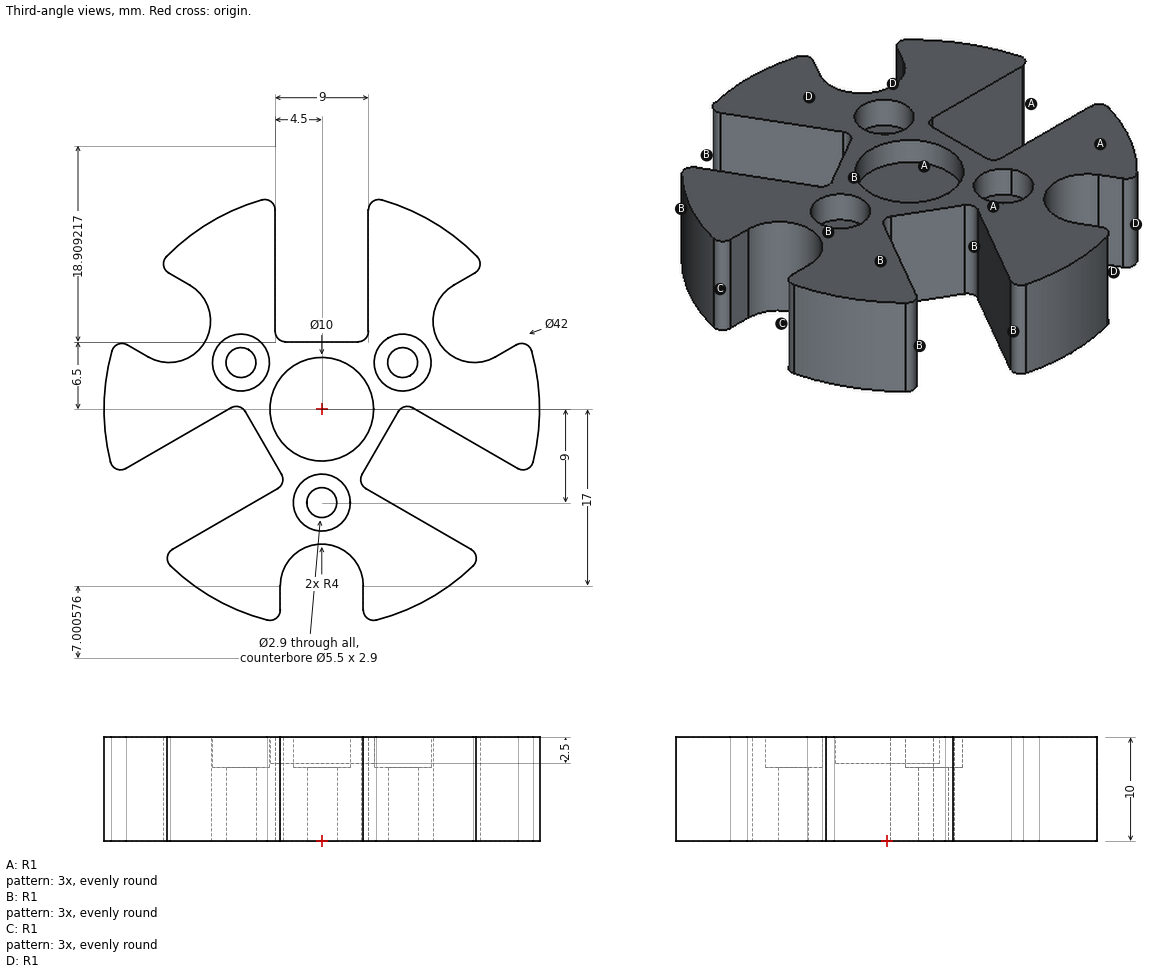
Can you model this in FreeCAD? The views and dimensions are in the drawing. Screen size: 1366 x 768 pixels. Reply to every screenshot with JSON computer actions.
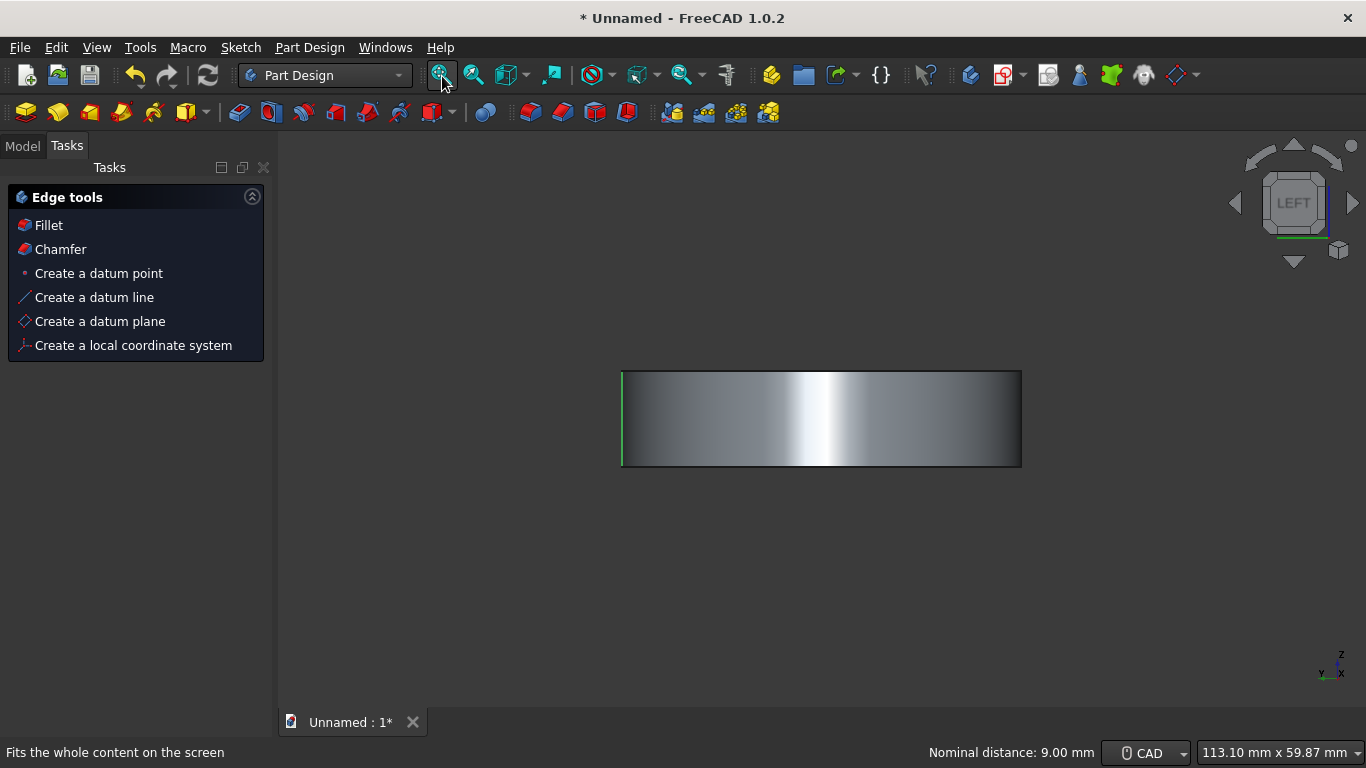
{"action": "key", "text": "v 3"}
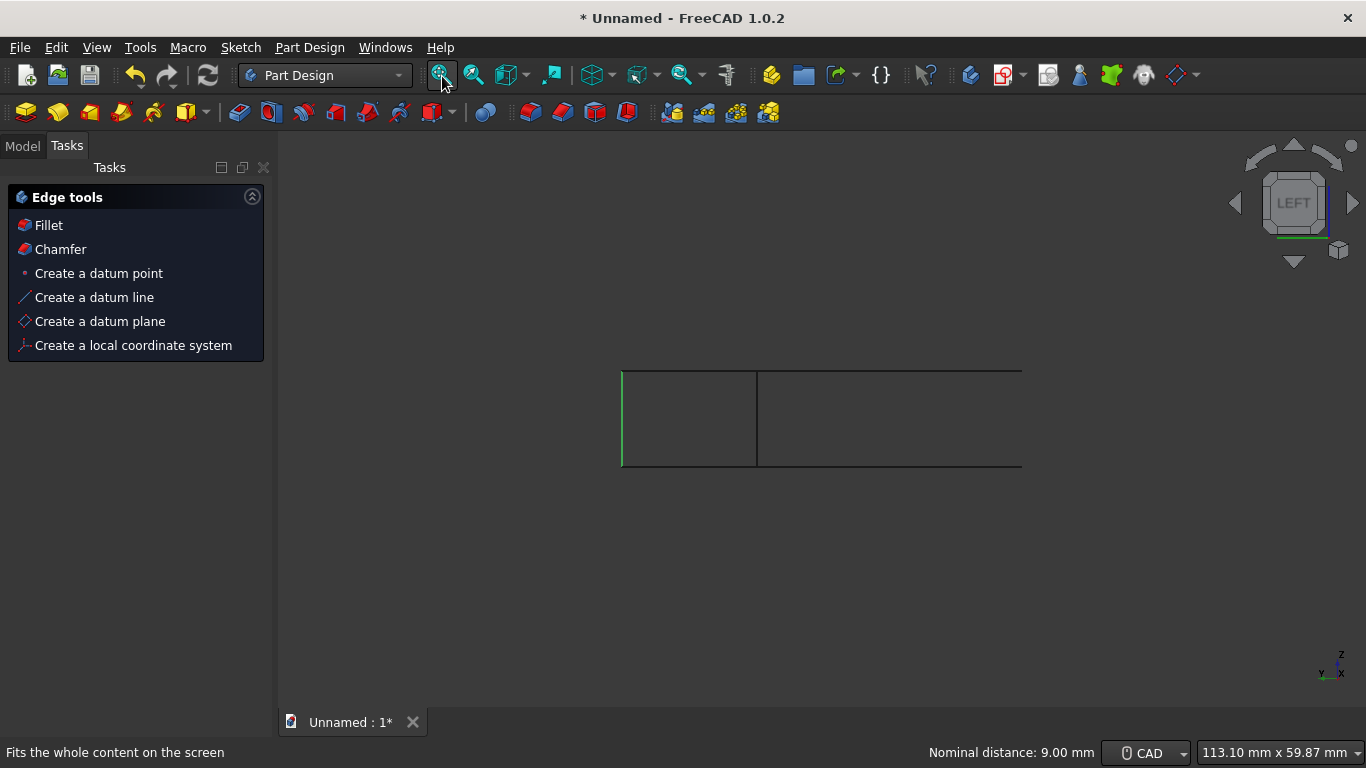
{"action": "key", "text": "0"}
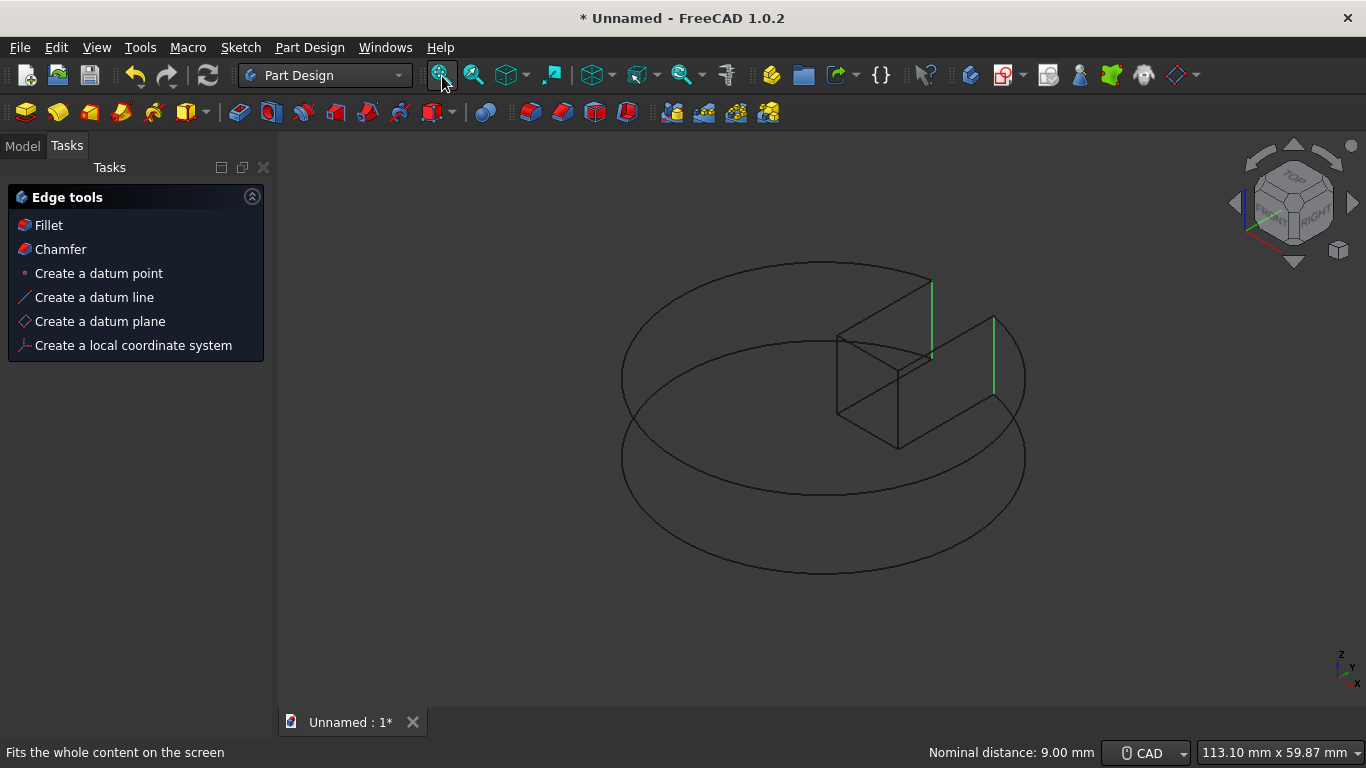
{"action": "left_click", "coordinate": [837, 374], "text": "ctrl"}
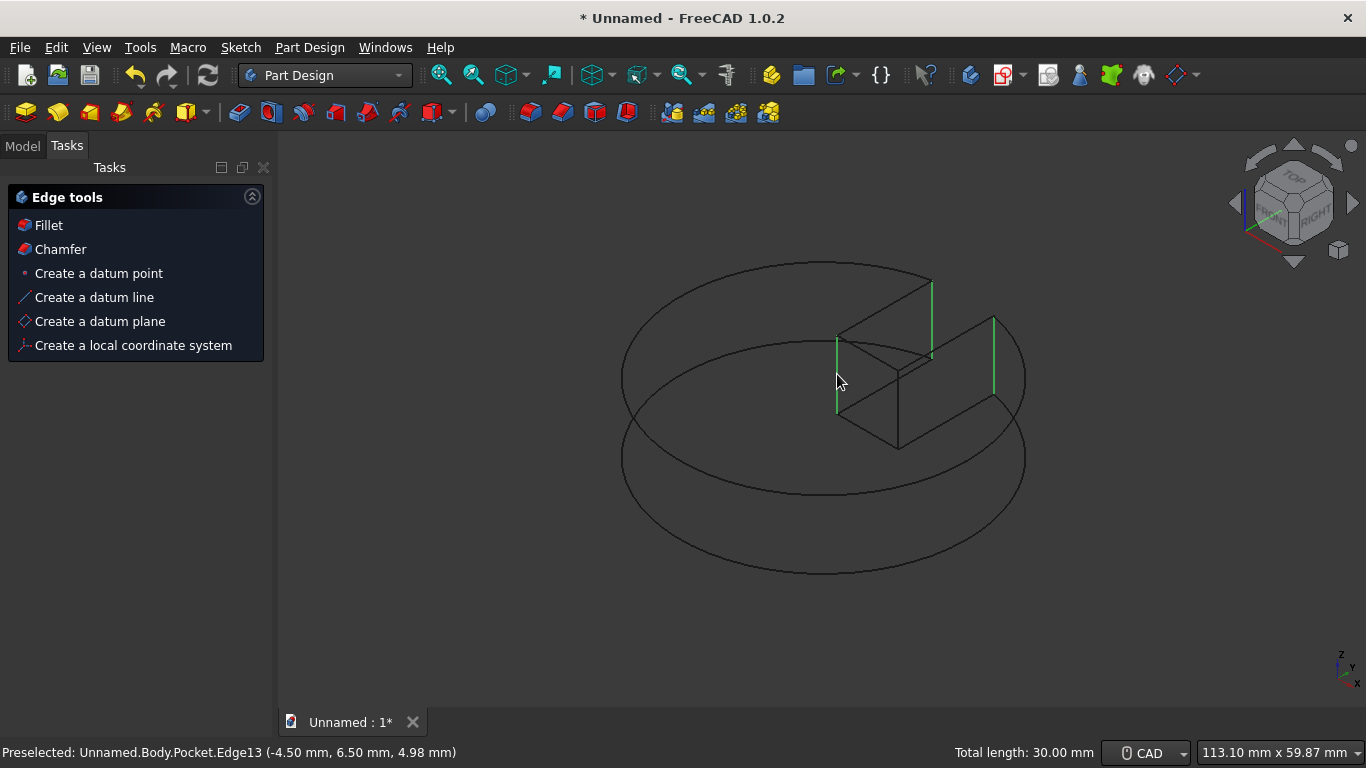
{"action": "left_click", "coordinate": [898, 409], "text": "ctrl"}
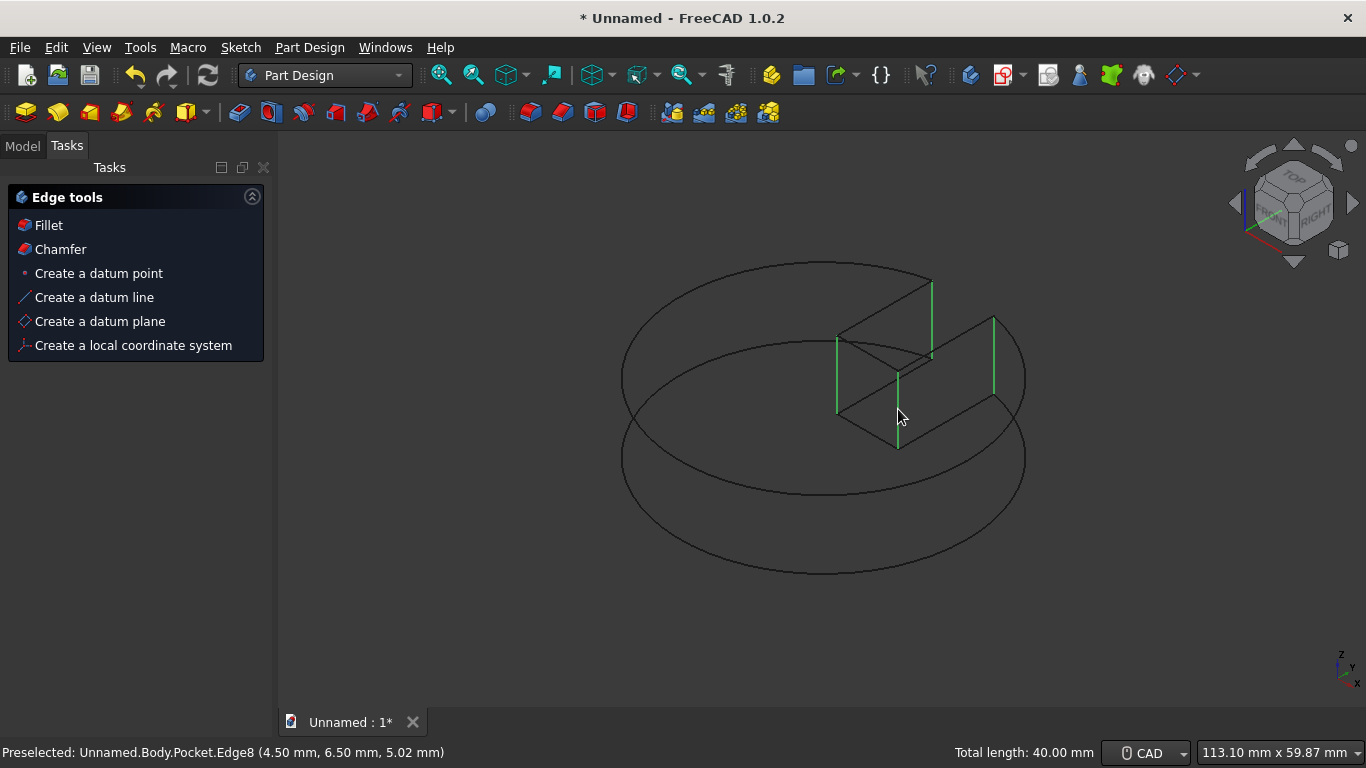
{"action": "key", "text": "v 1"}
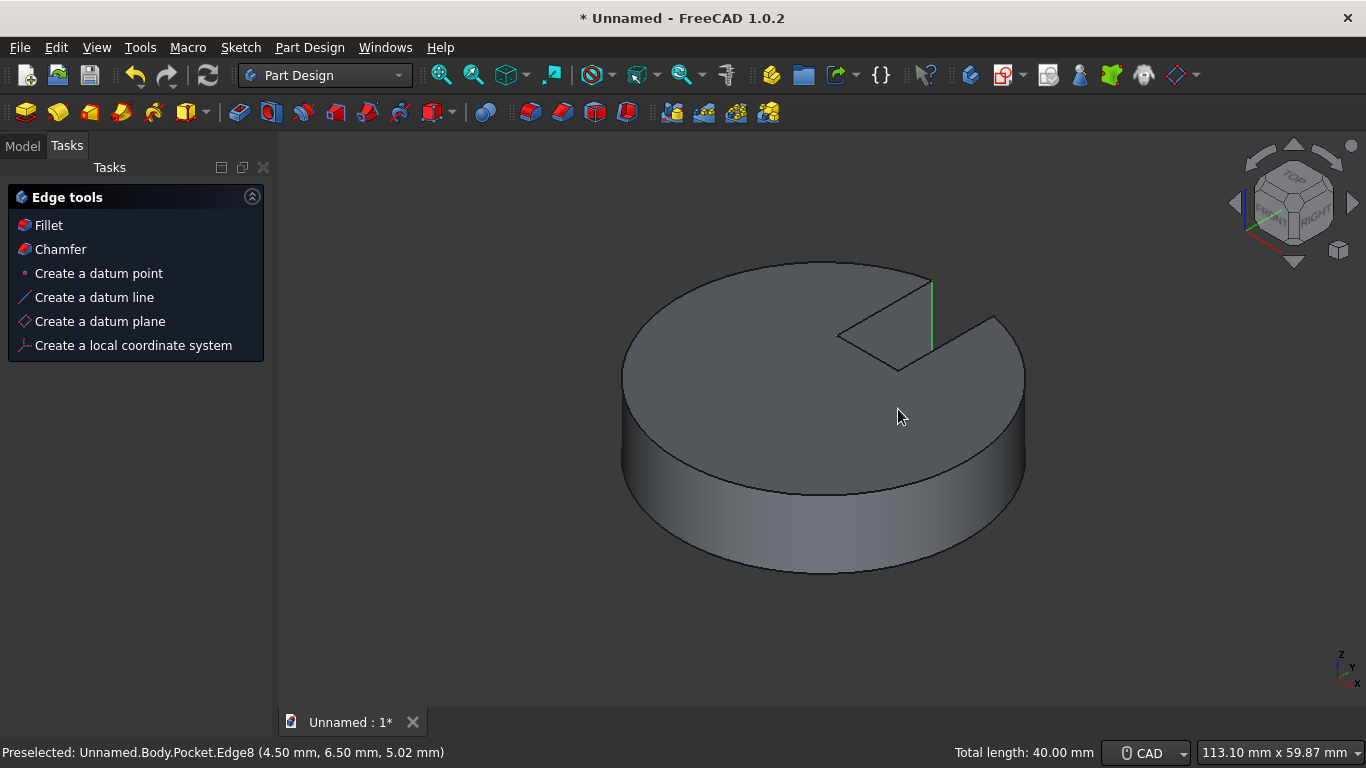
{"action": "left_click", "coordinate": [532, 112]}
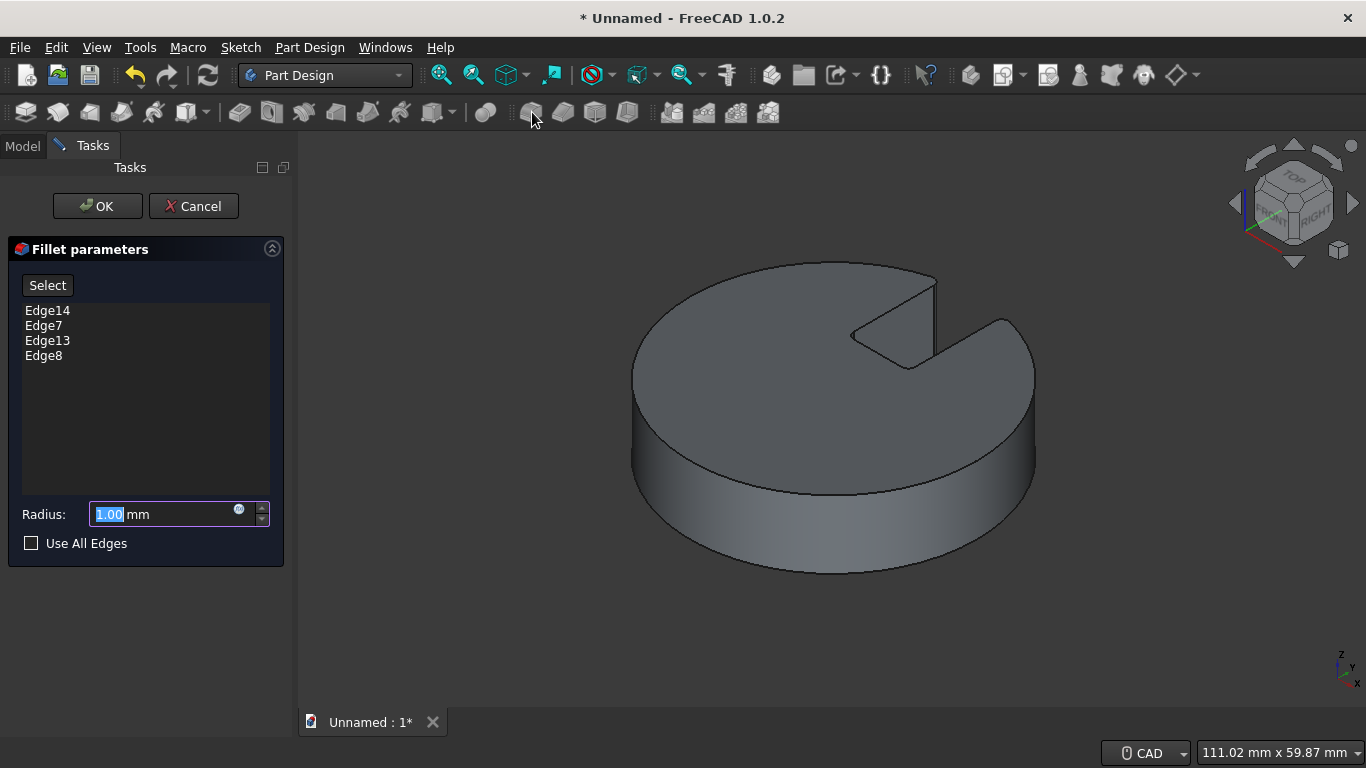
{"action": "type", "text": "1"}
{"action": "key", "text": "Tab"}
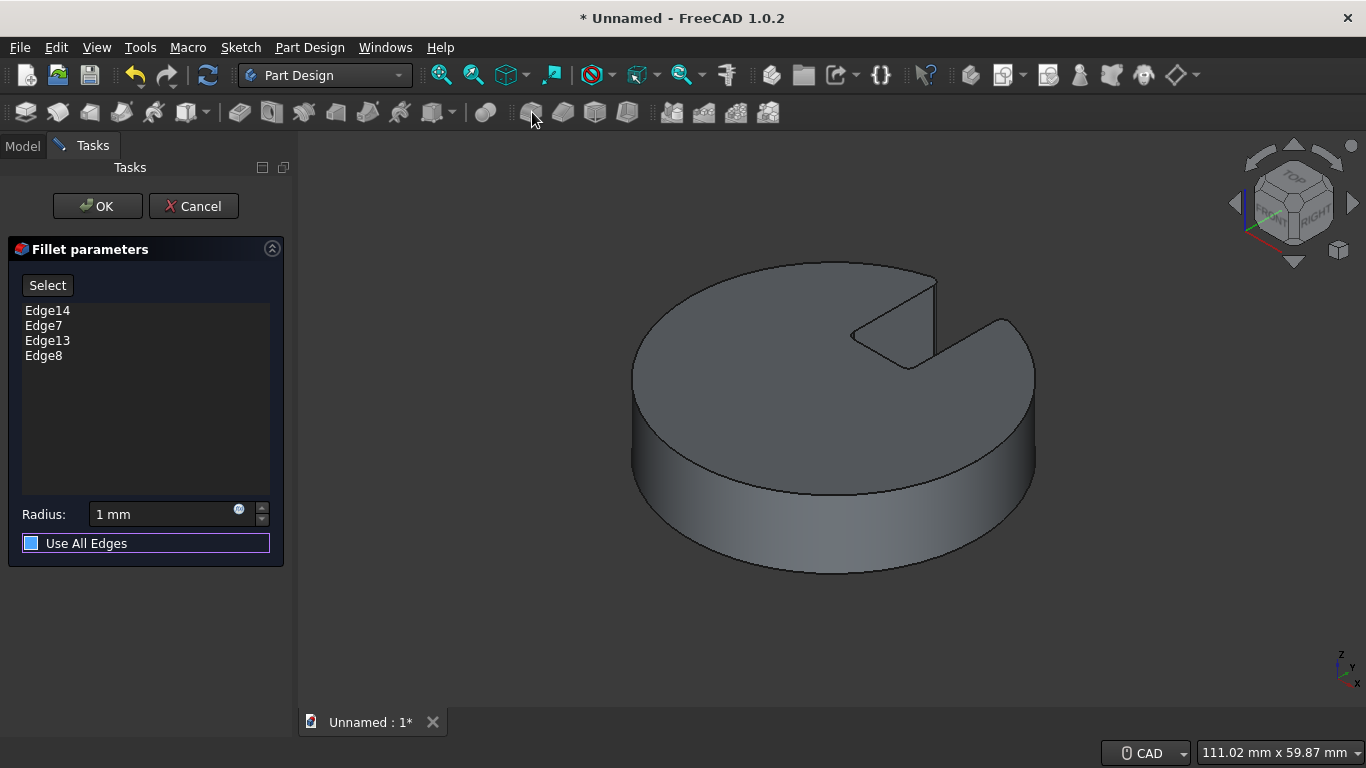
{"action": "left_click", "coordinate": [98, 206]}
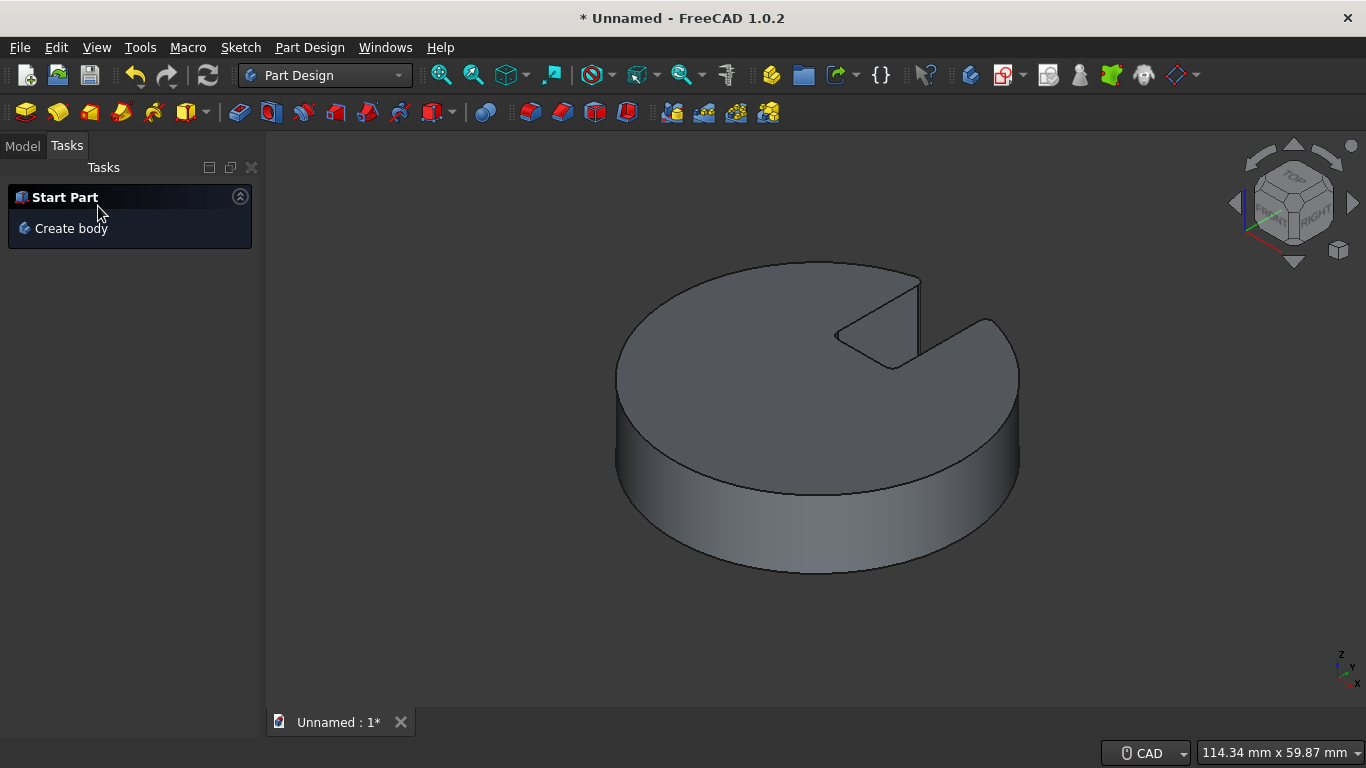
{"action": "left_click", "coordinate": [23, 145]}